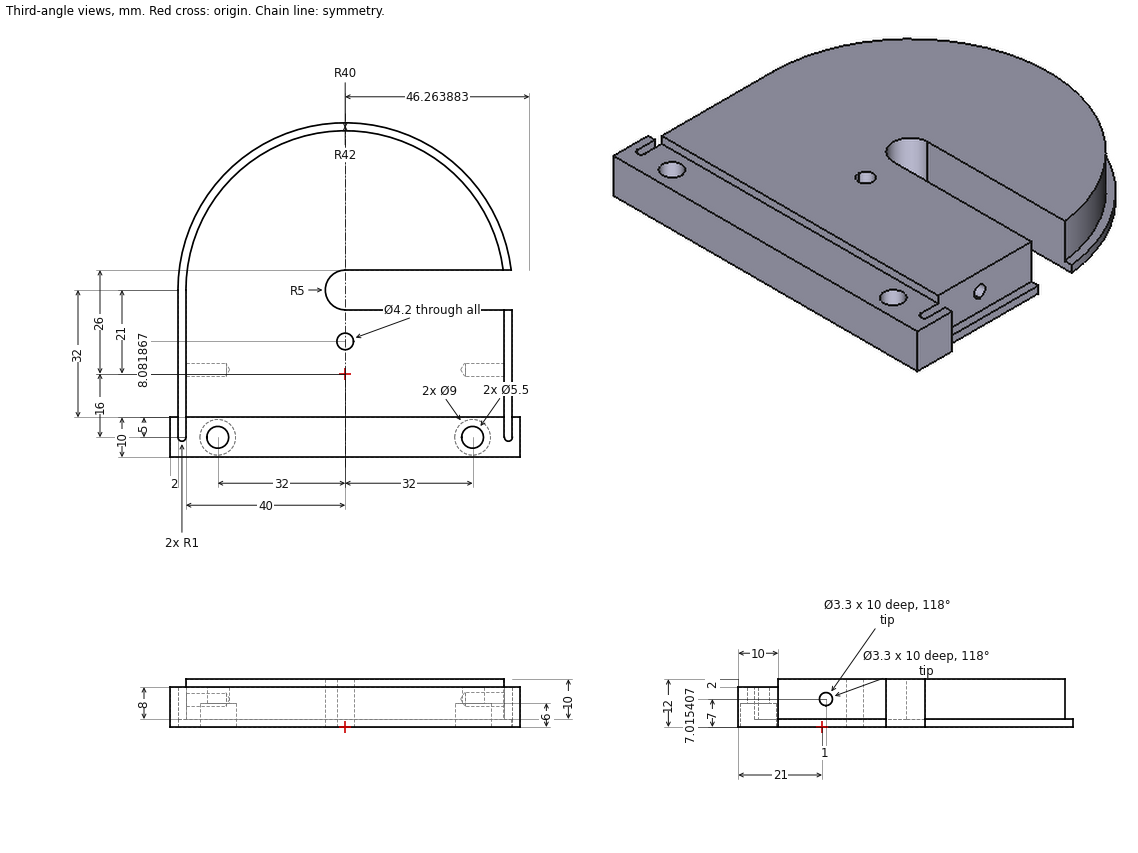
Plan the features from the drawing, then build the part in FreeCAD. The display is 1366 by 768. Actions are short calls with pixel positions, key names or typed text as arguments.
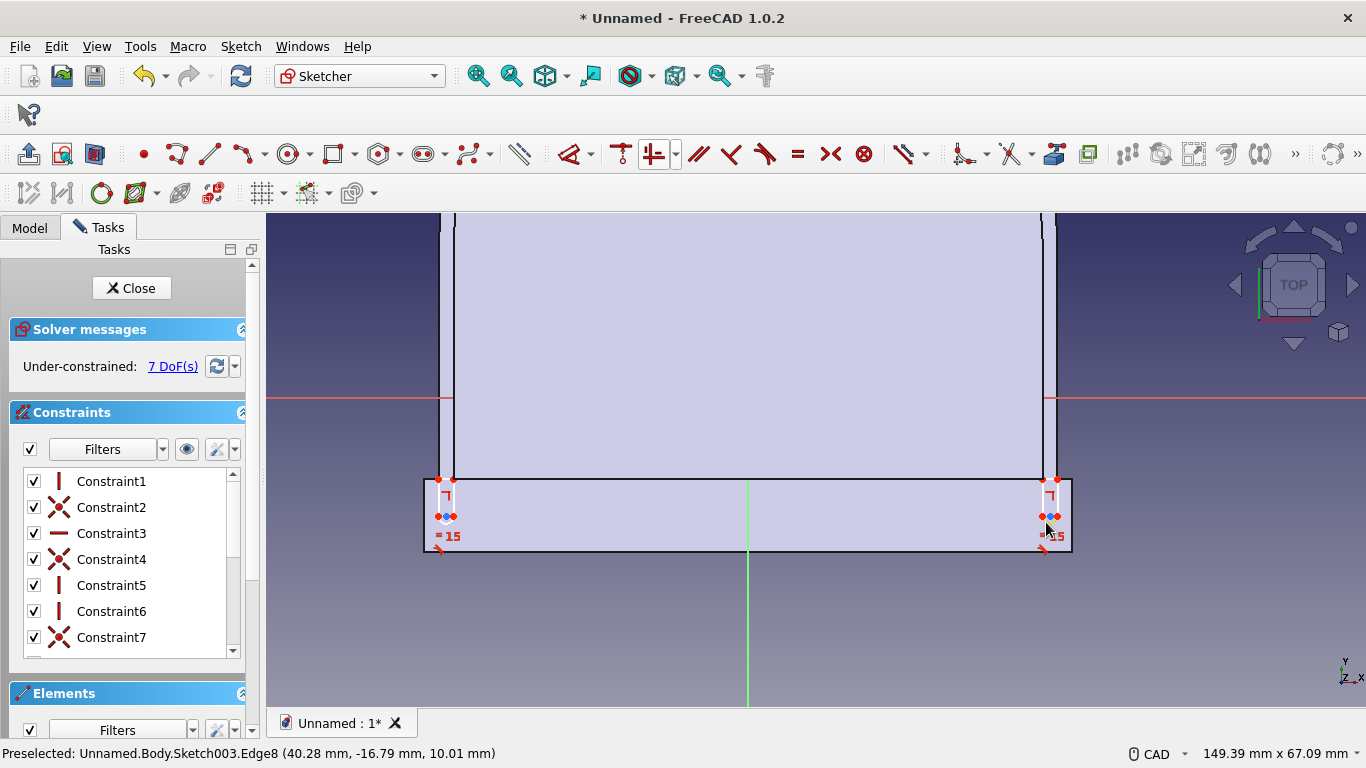
scroll(446, 516, up, 3)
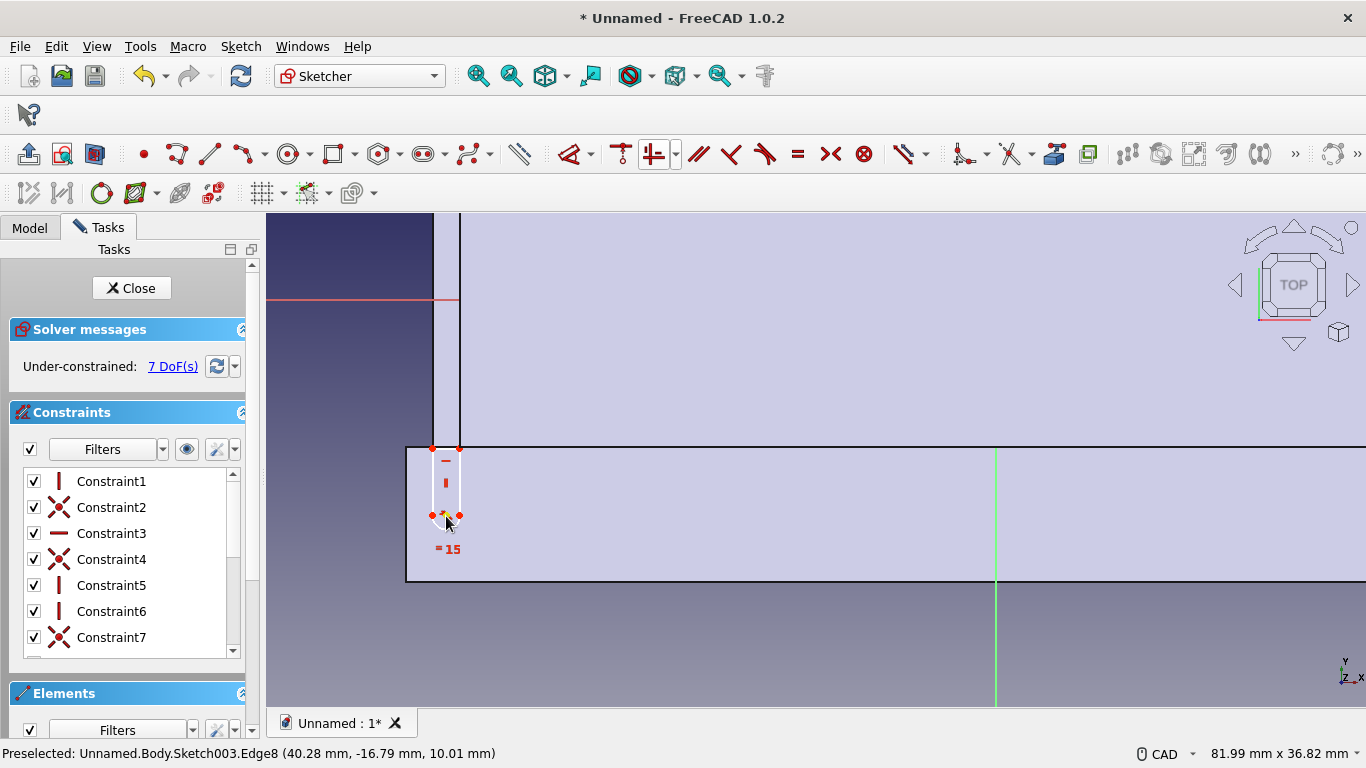
click(446, 516)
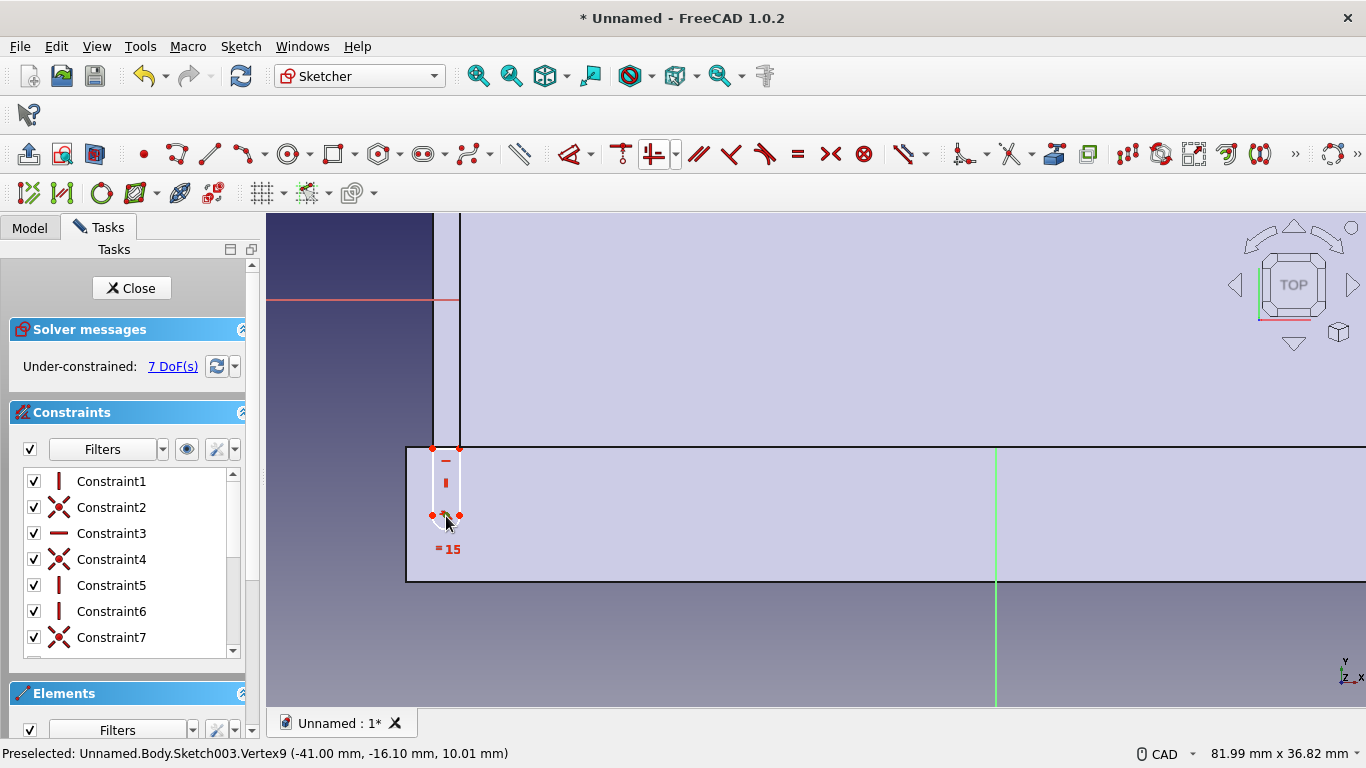
scroll(445, 516, down, 3)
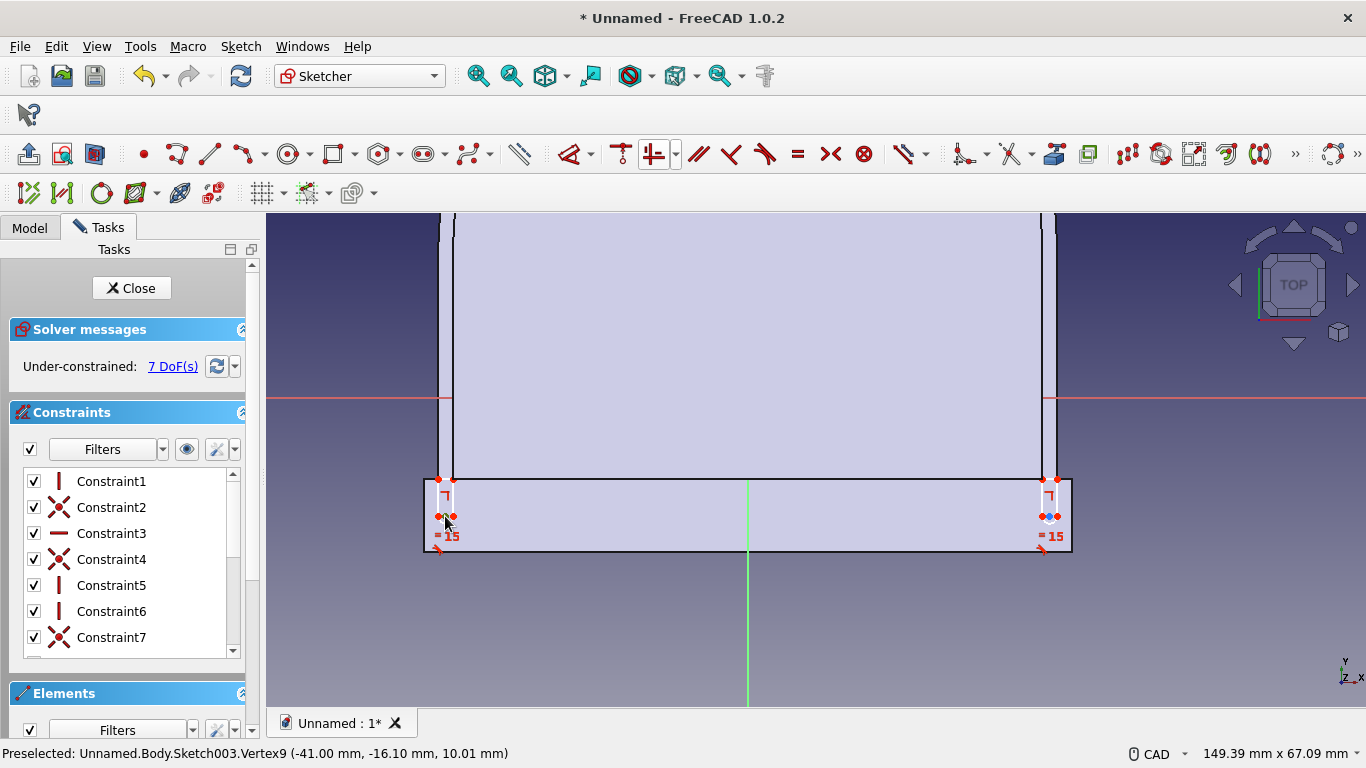
scroll(1050, 516, up, 3)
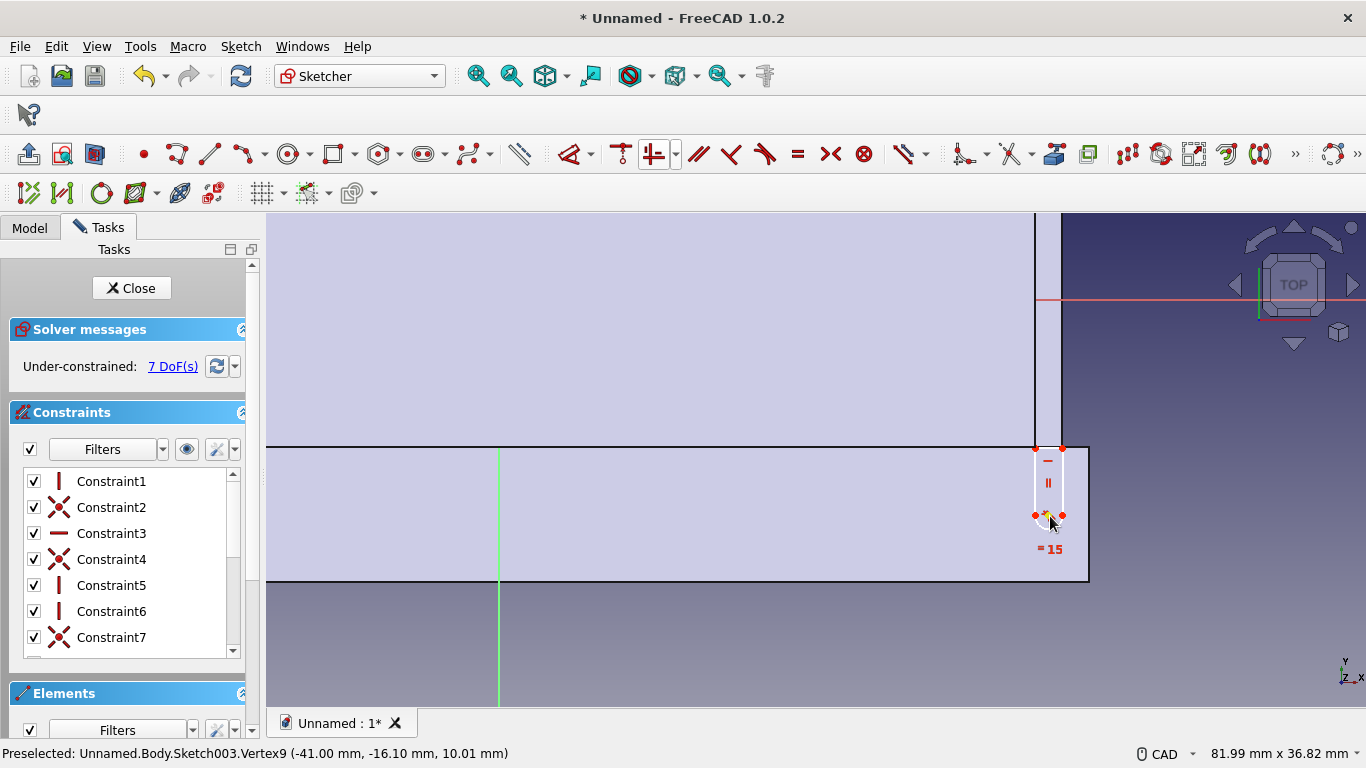
click(1049, 516)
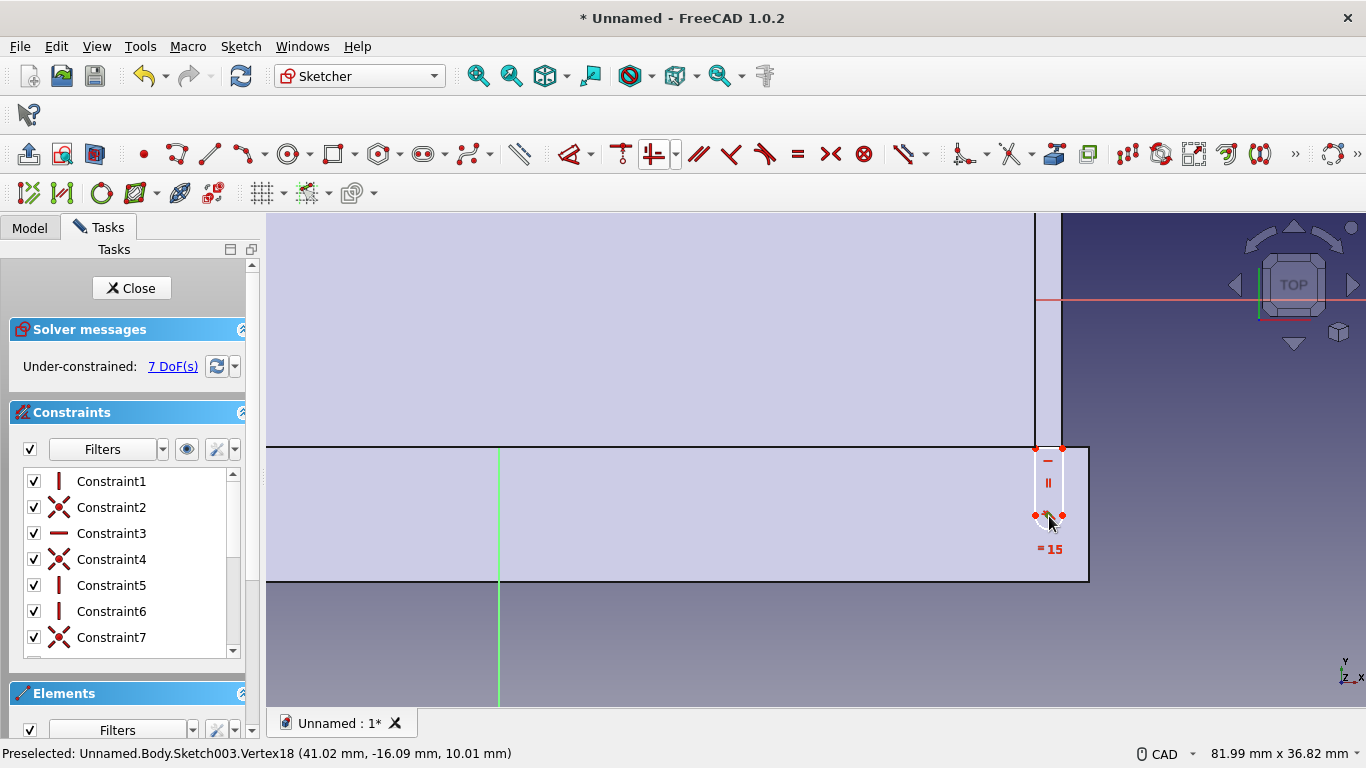
click(499, 648)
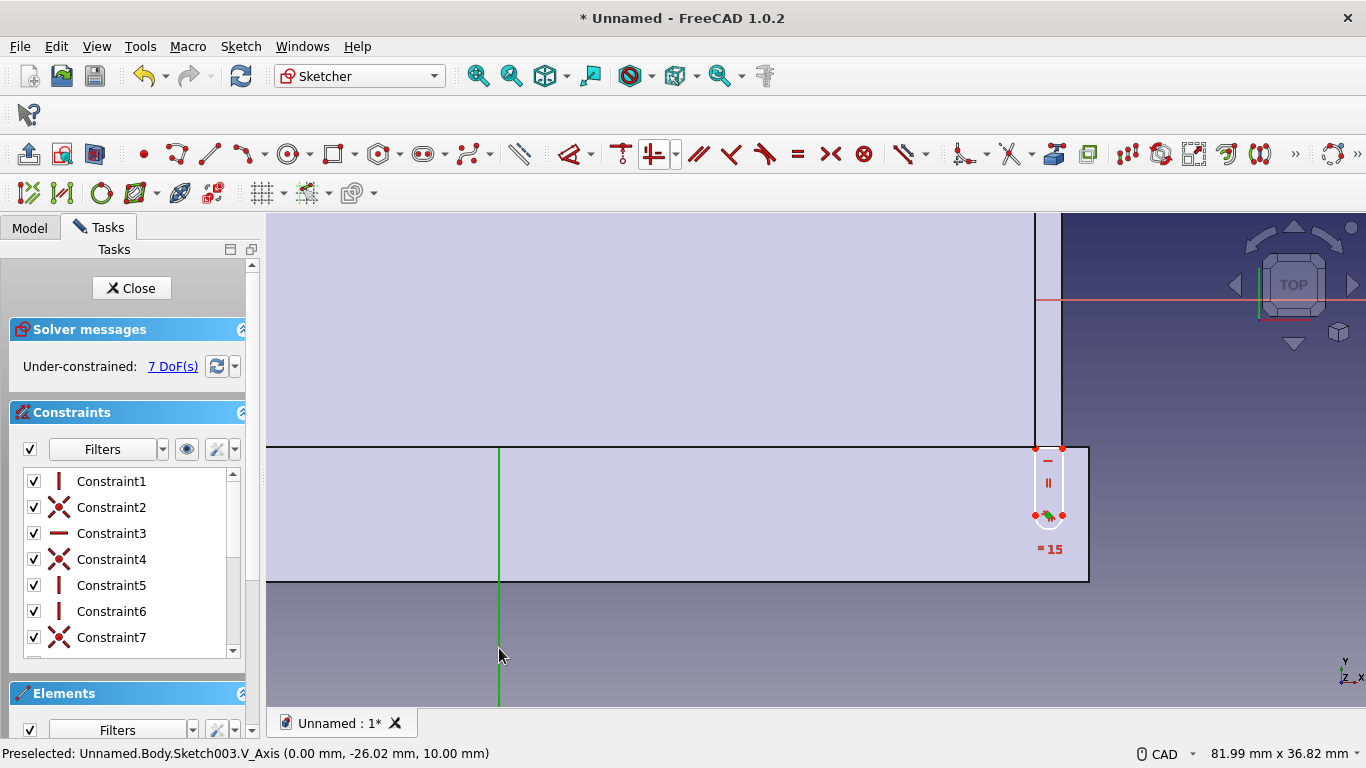
click(831, 154)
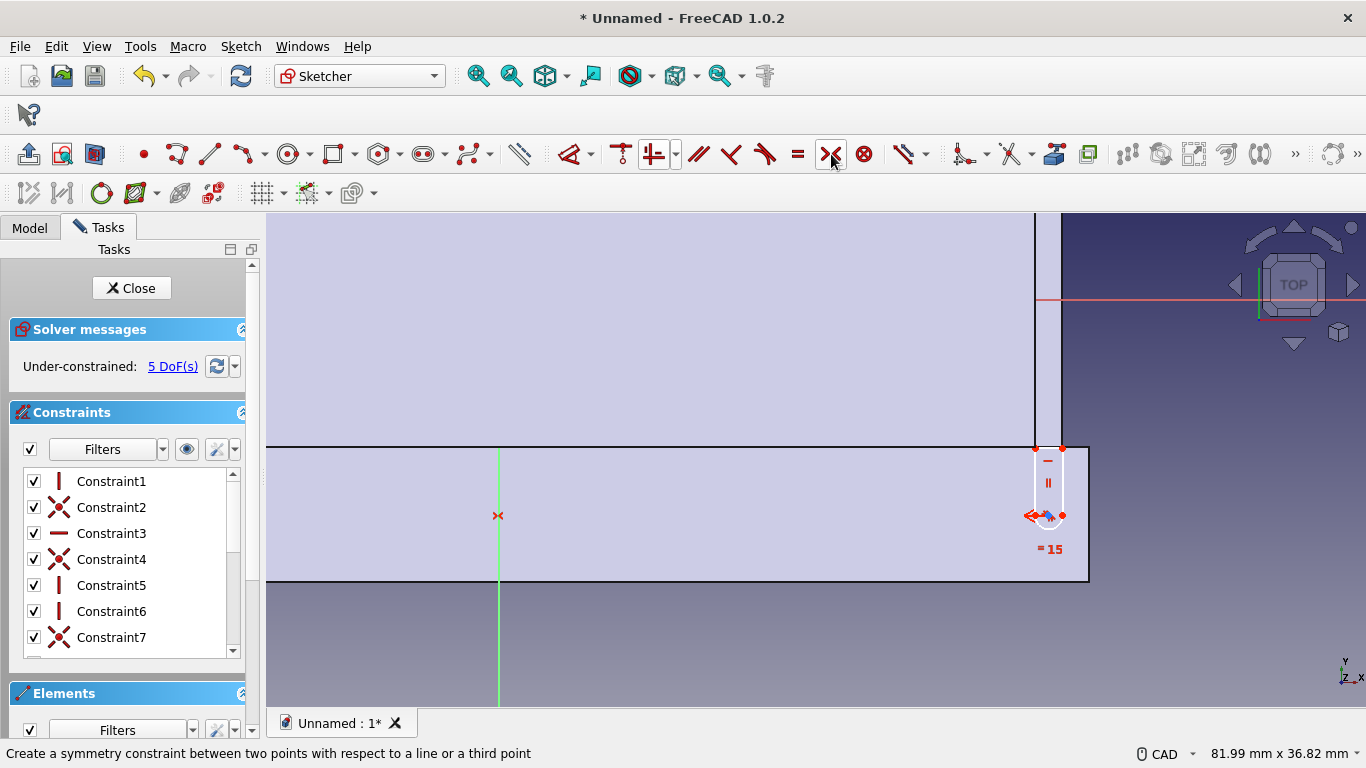
click(568, 154)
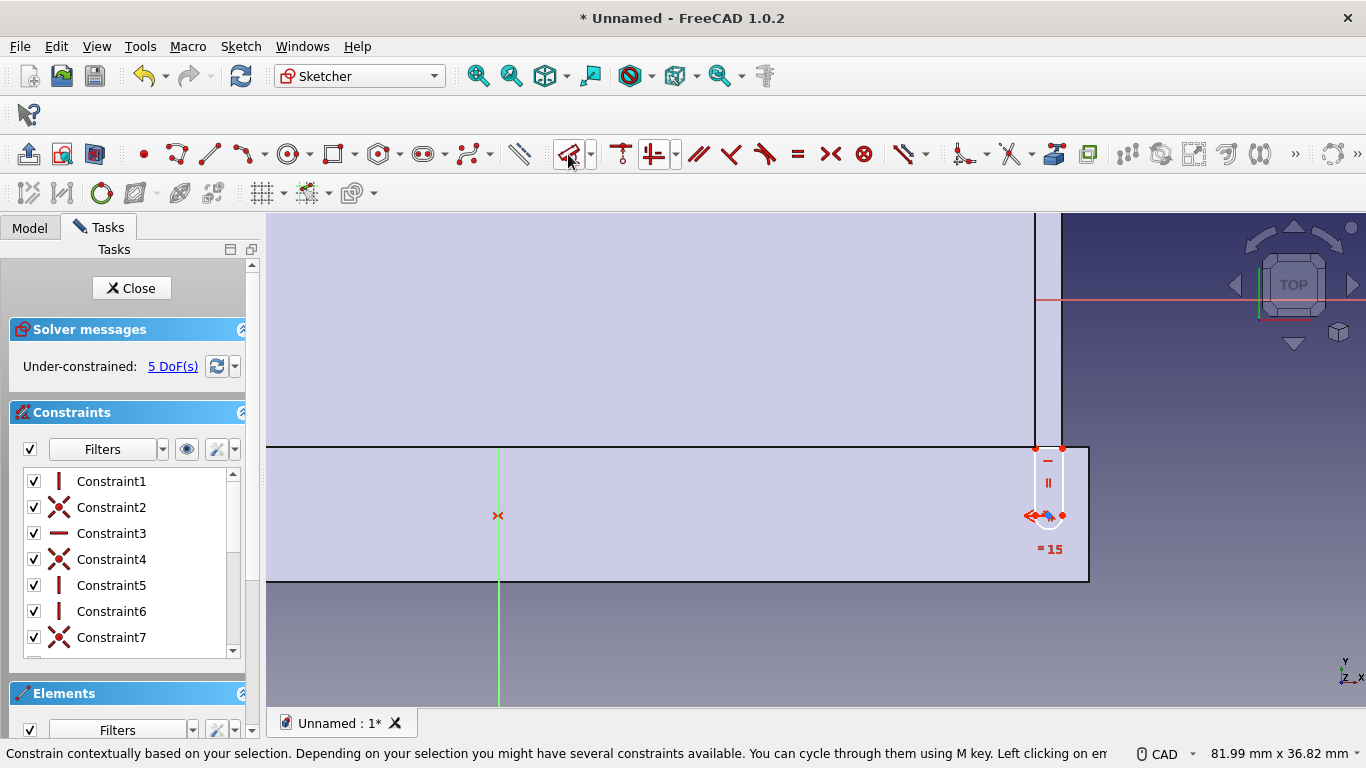
scroll(1050, 516, down, 3)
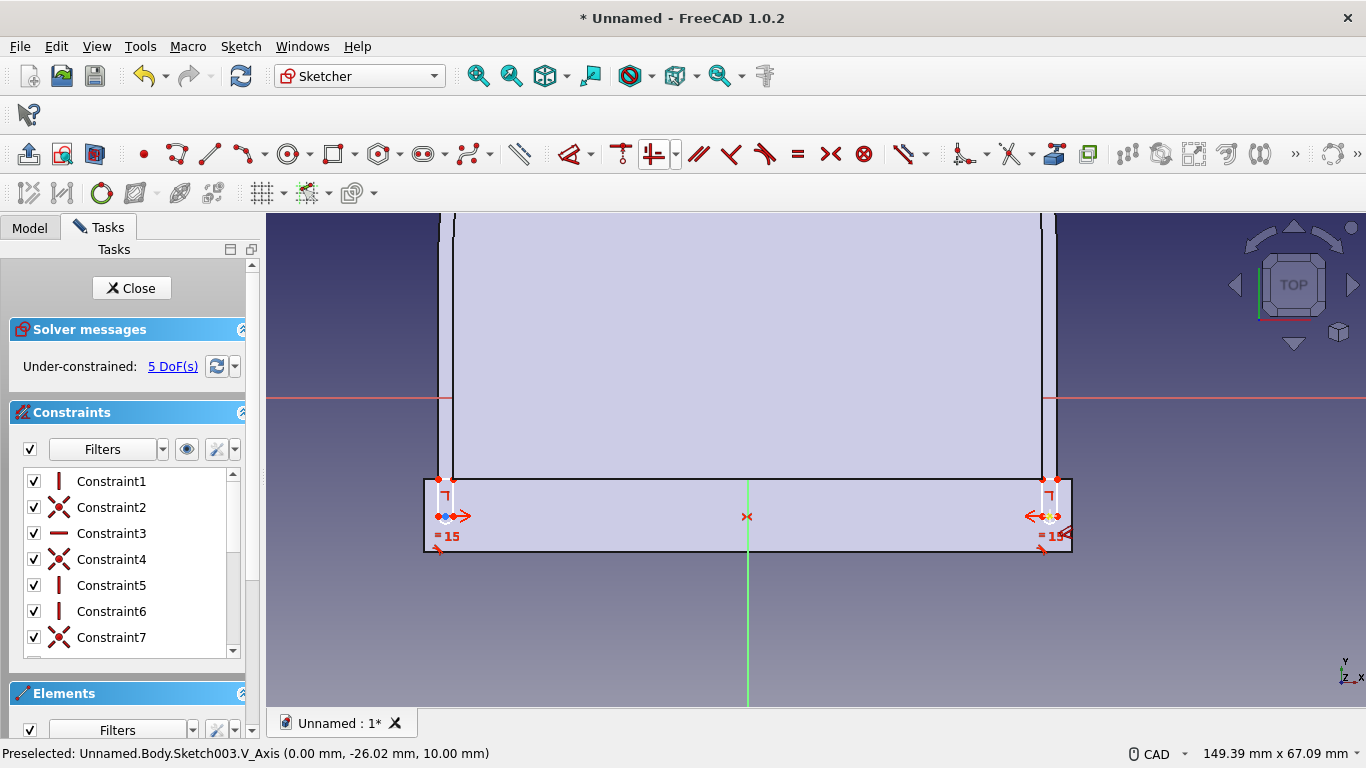
scroll(441, 522, up, 9)